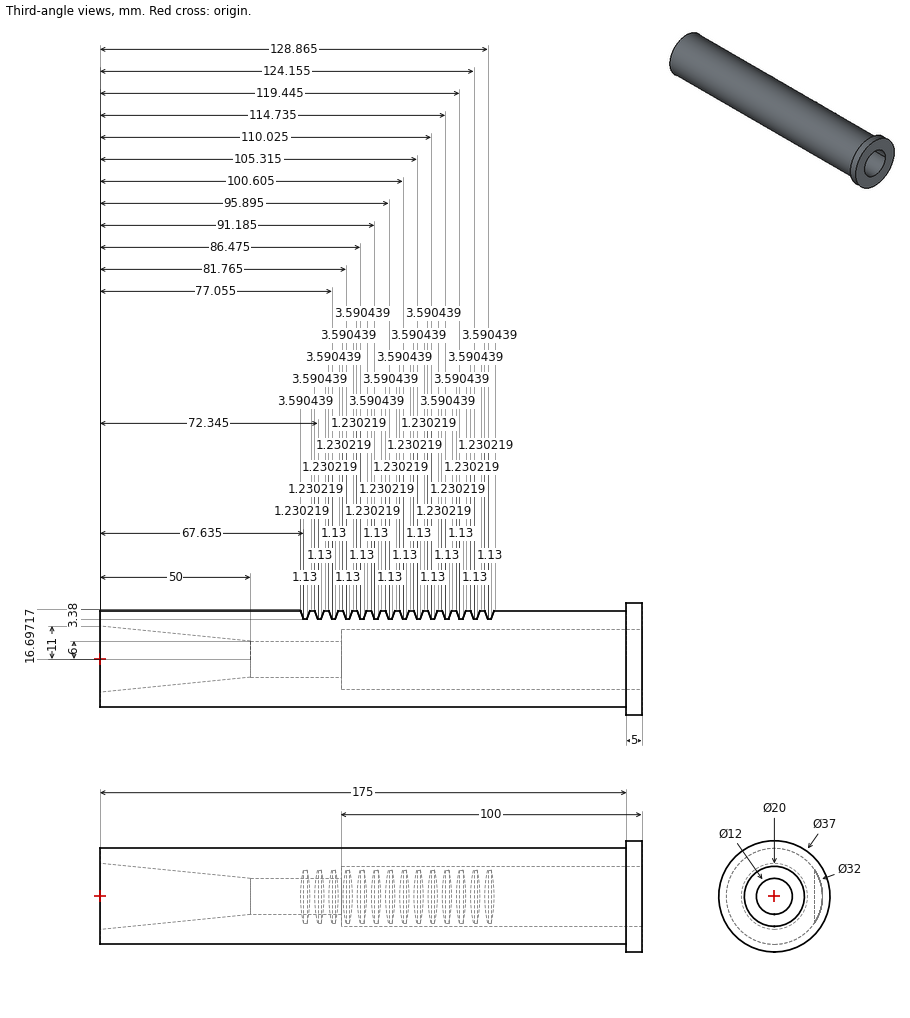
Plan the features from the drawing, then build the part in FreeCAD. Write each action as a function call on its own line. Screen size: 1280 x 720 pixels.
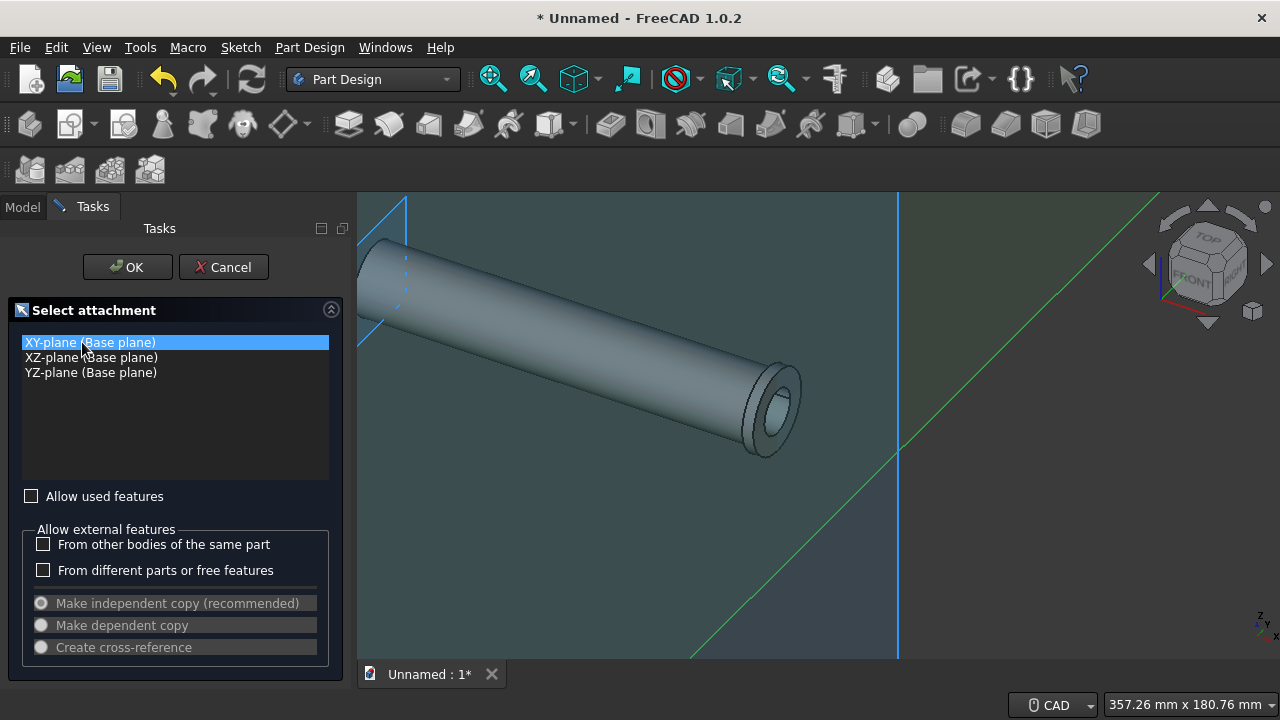
click(128, 267)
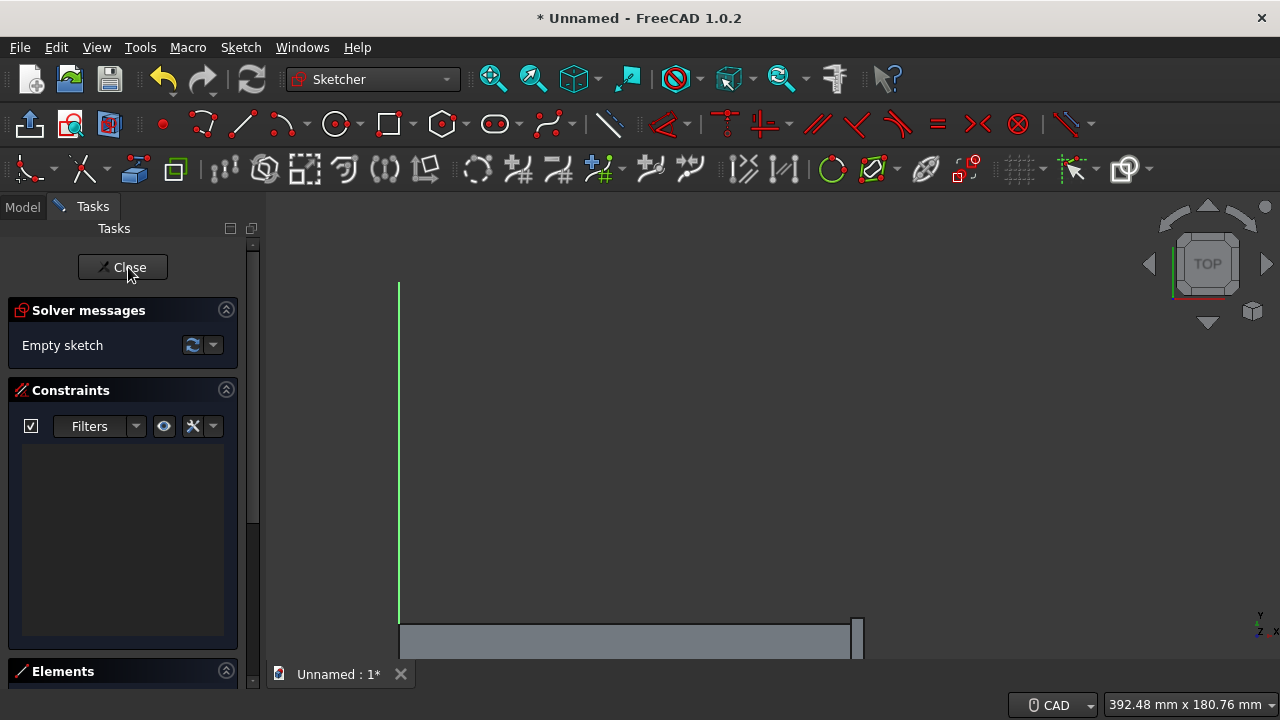
click(110, 124)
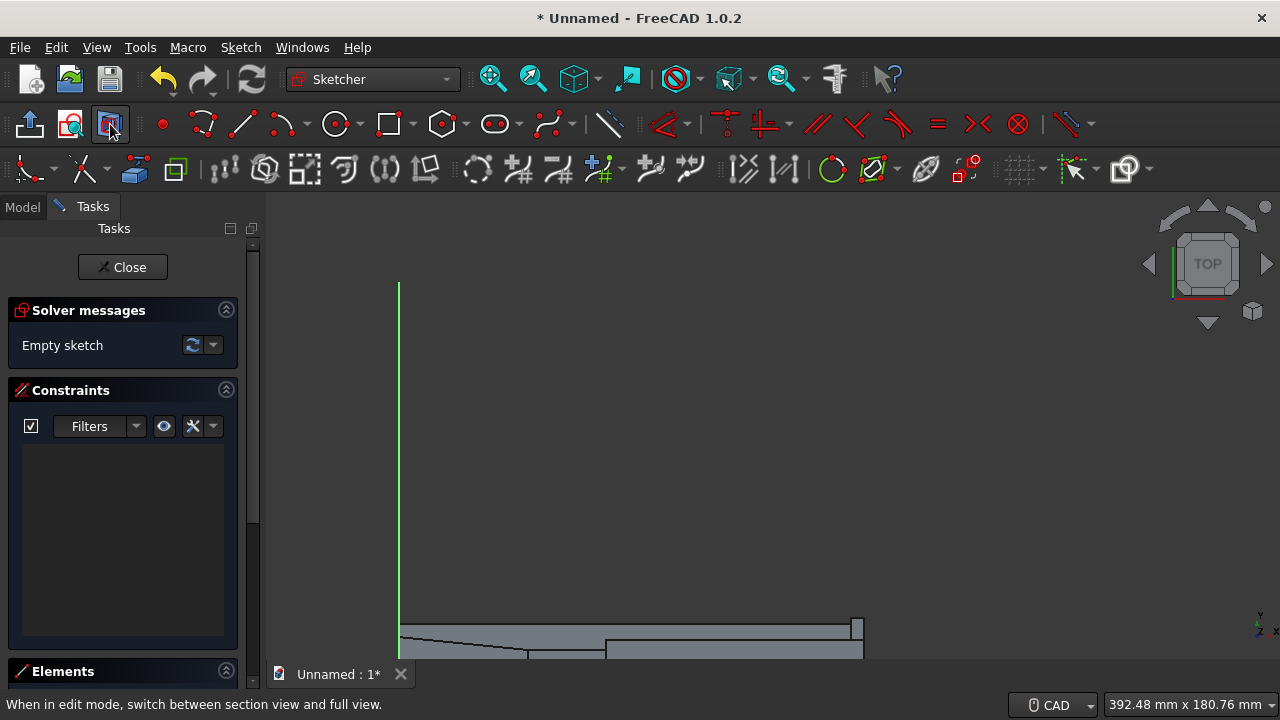
scroll(704, 426, down, 5)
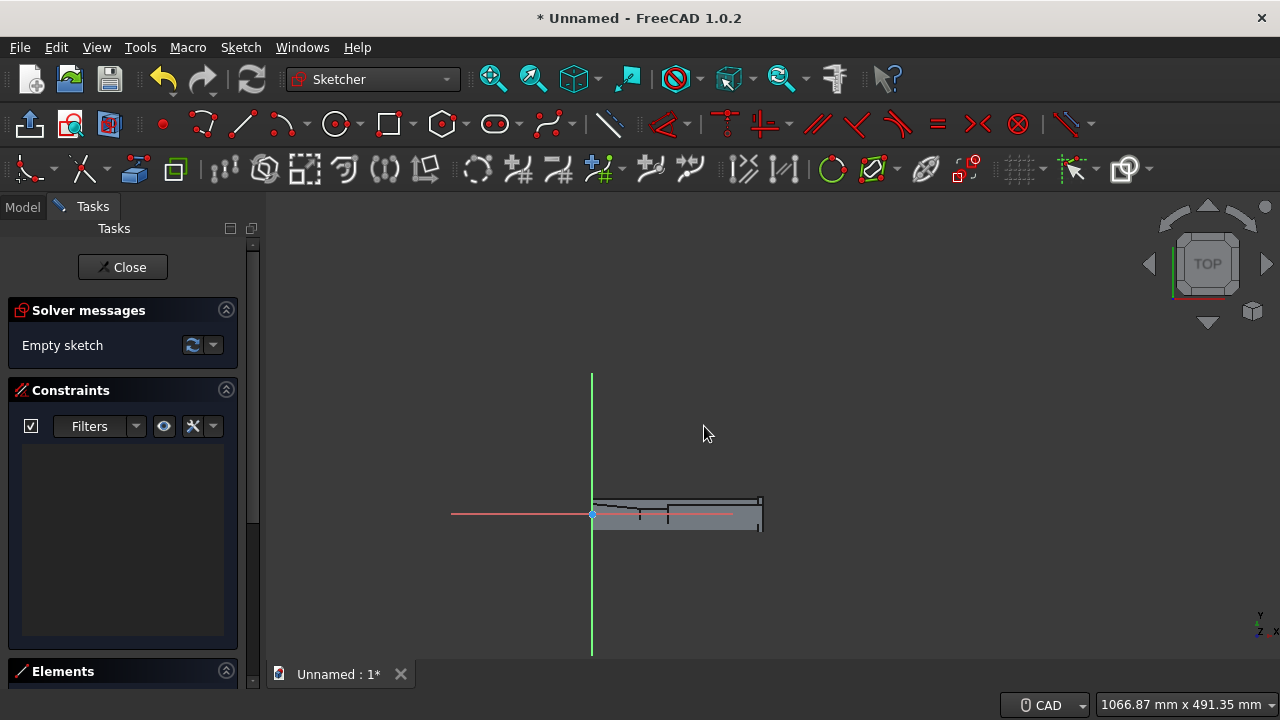
scroll(642, 527, up, 8)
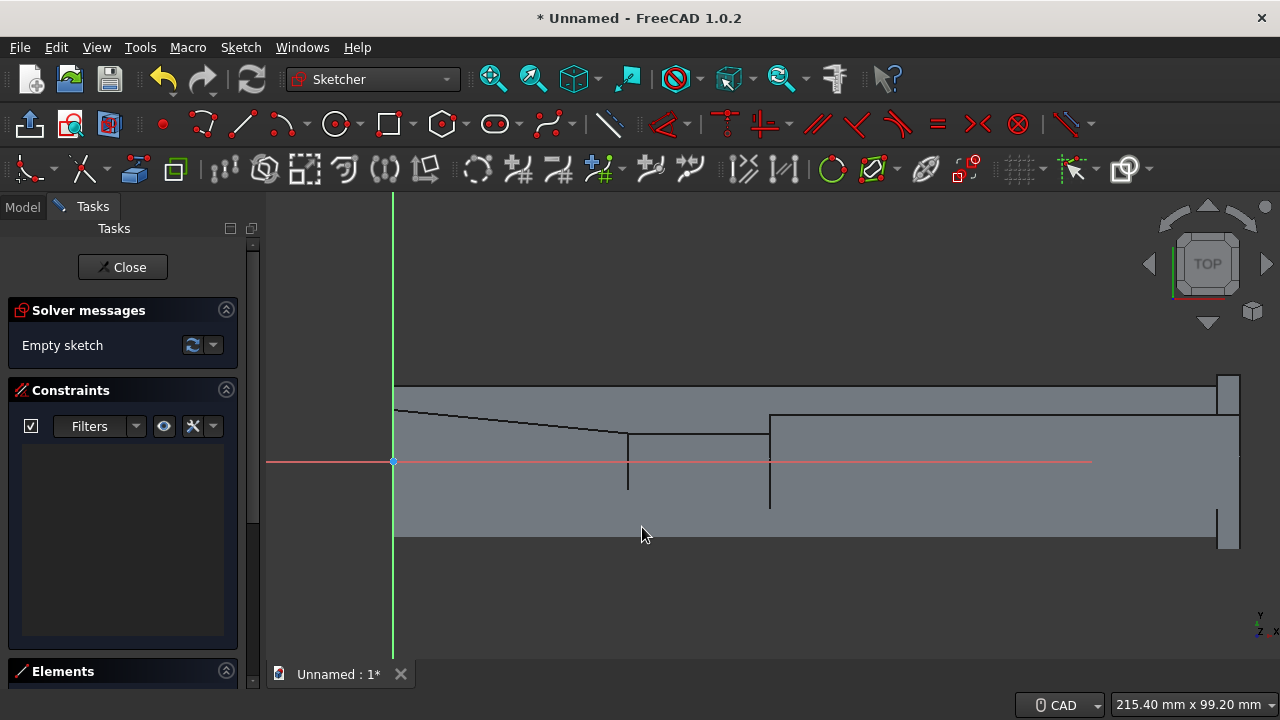
key(g)
key(m)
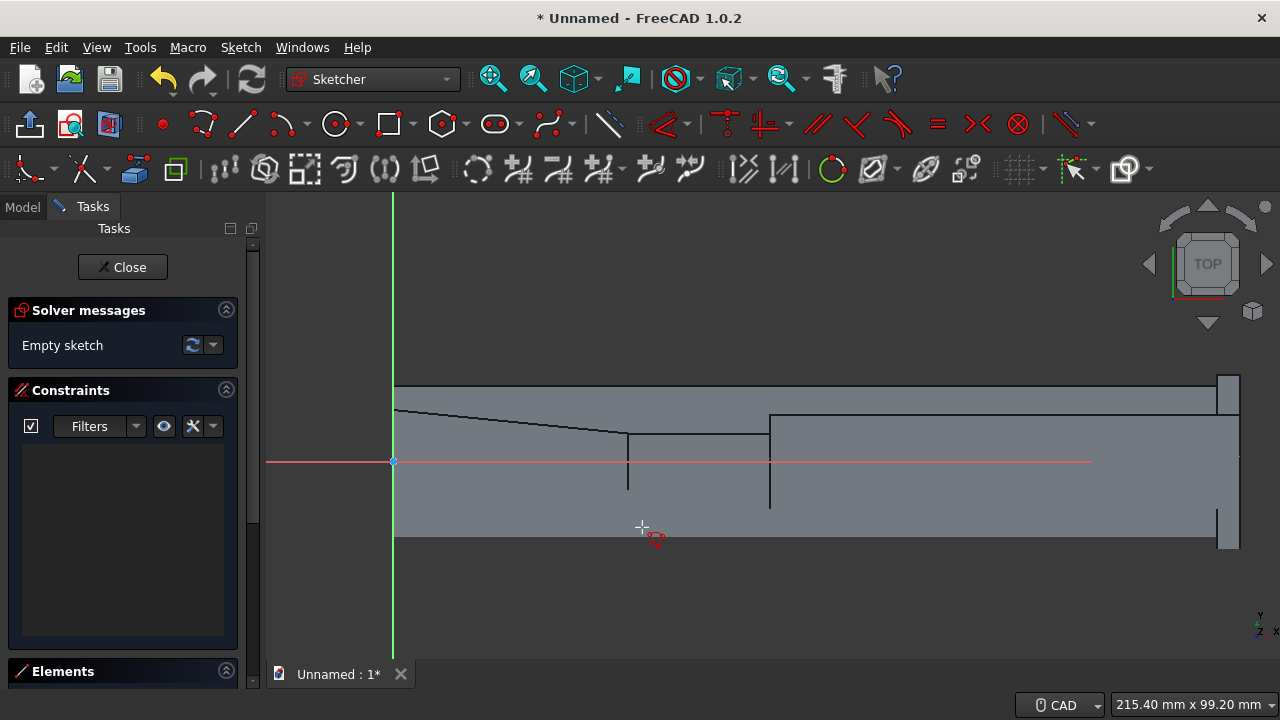
click(706, 383)
click(711, 399)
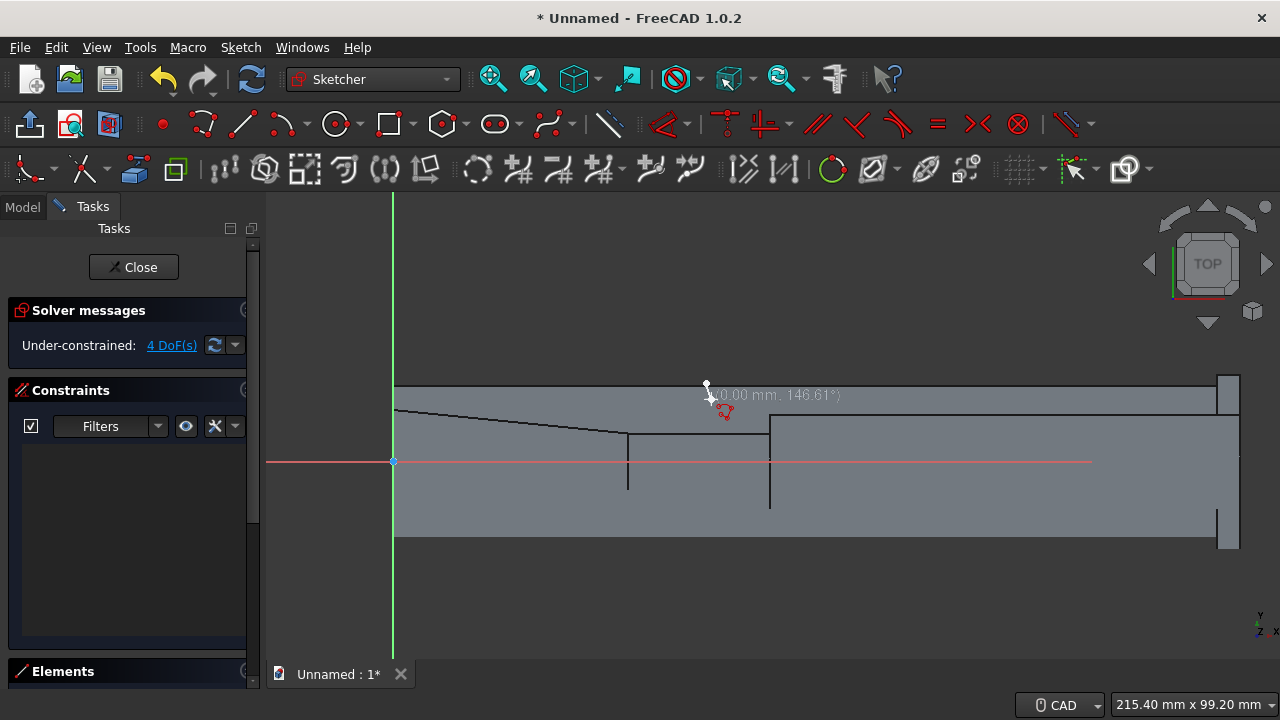
scroll(717, 399, up, 6)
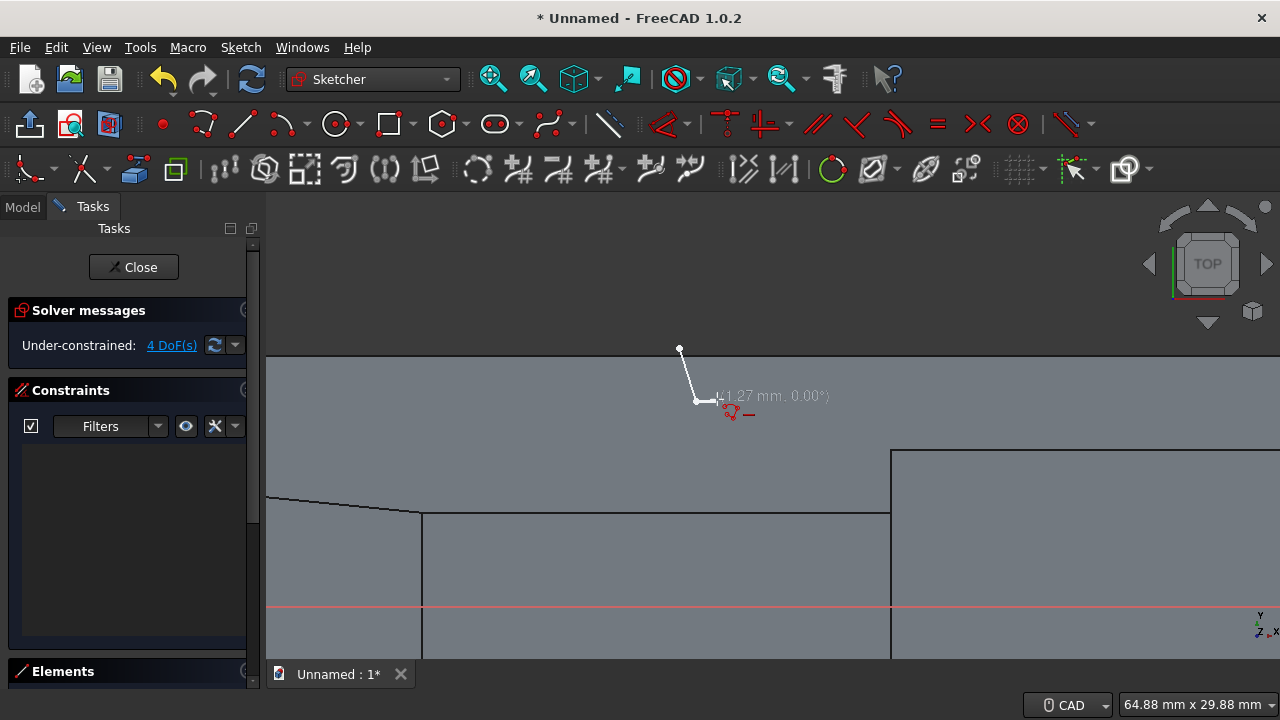
click(715, 398)
click(735, 346)
click(679, 348)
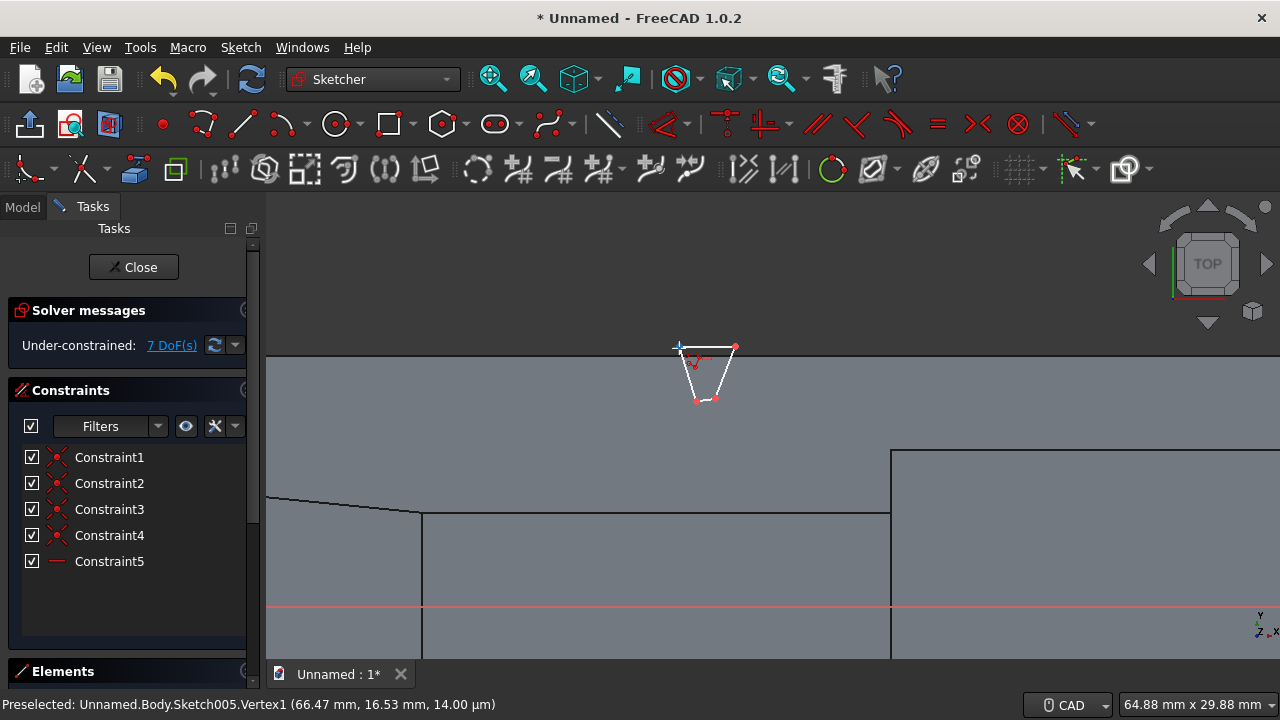
click(752, 346)
click(771, 398)
click(789, 398)
click(808, 346)
click(752, 347)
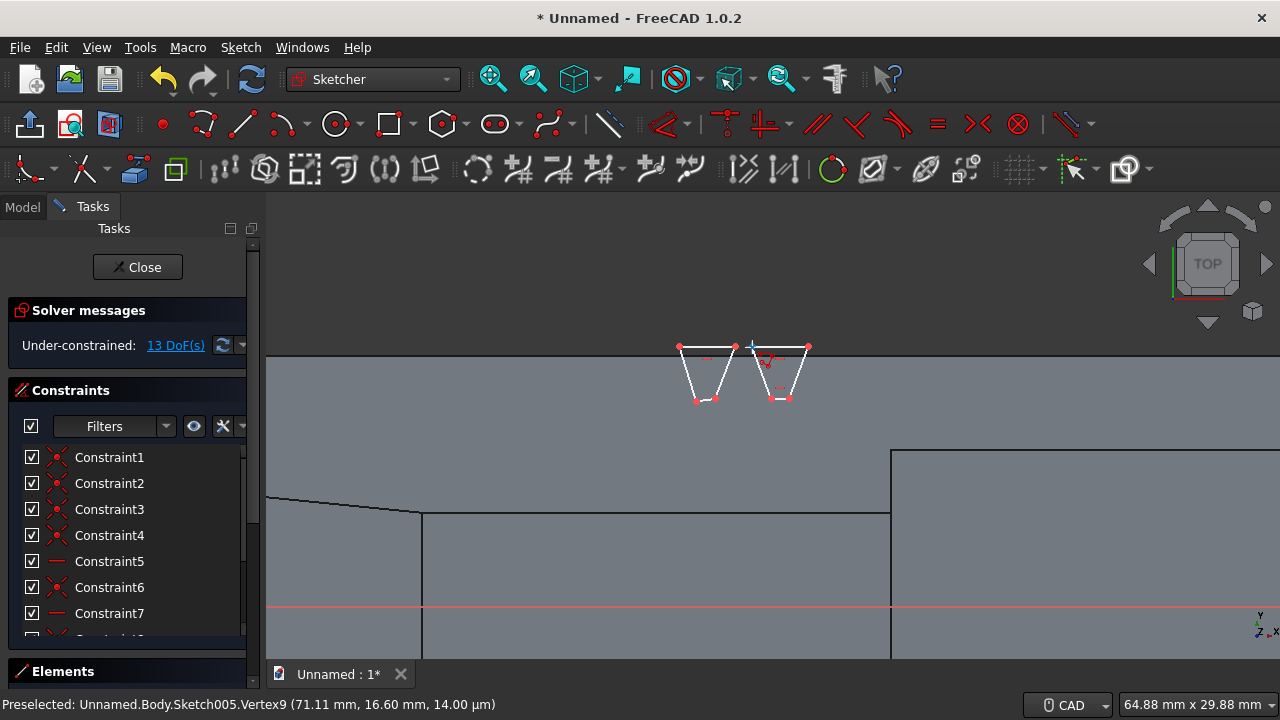
click(826, 346)
click(845, 398)
click(863, 398)
click(882, 346)
click(826, 347)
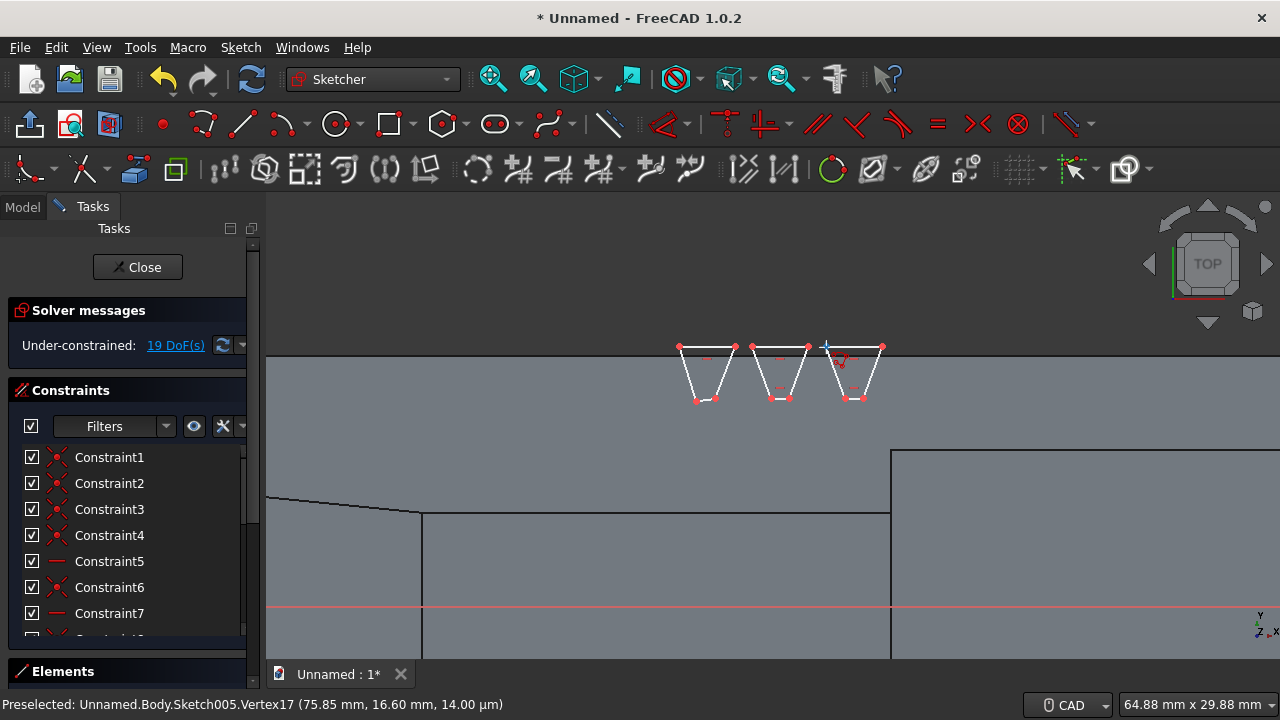
click(899, 346)
click(918, 398)
click(936, 398)
click(955, 346)
click(899, 347)